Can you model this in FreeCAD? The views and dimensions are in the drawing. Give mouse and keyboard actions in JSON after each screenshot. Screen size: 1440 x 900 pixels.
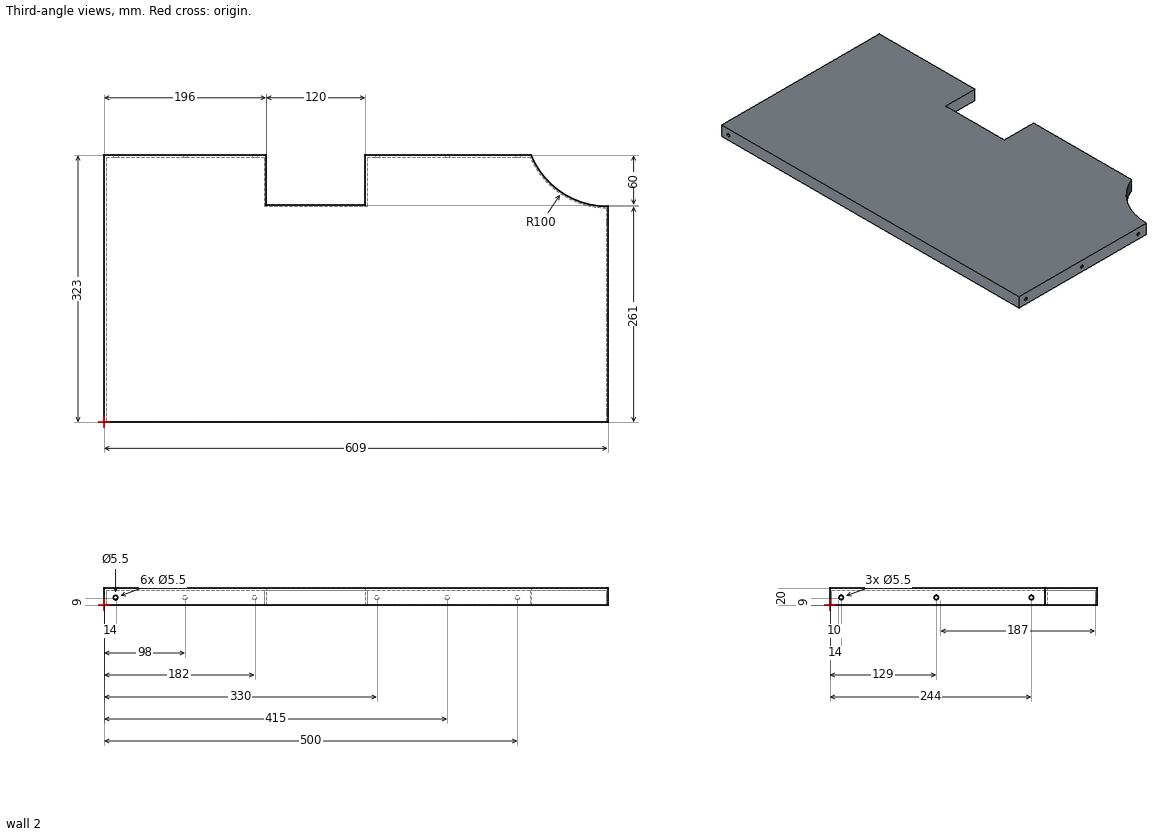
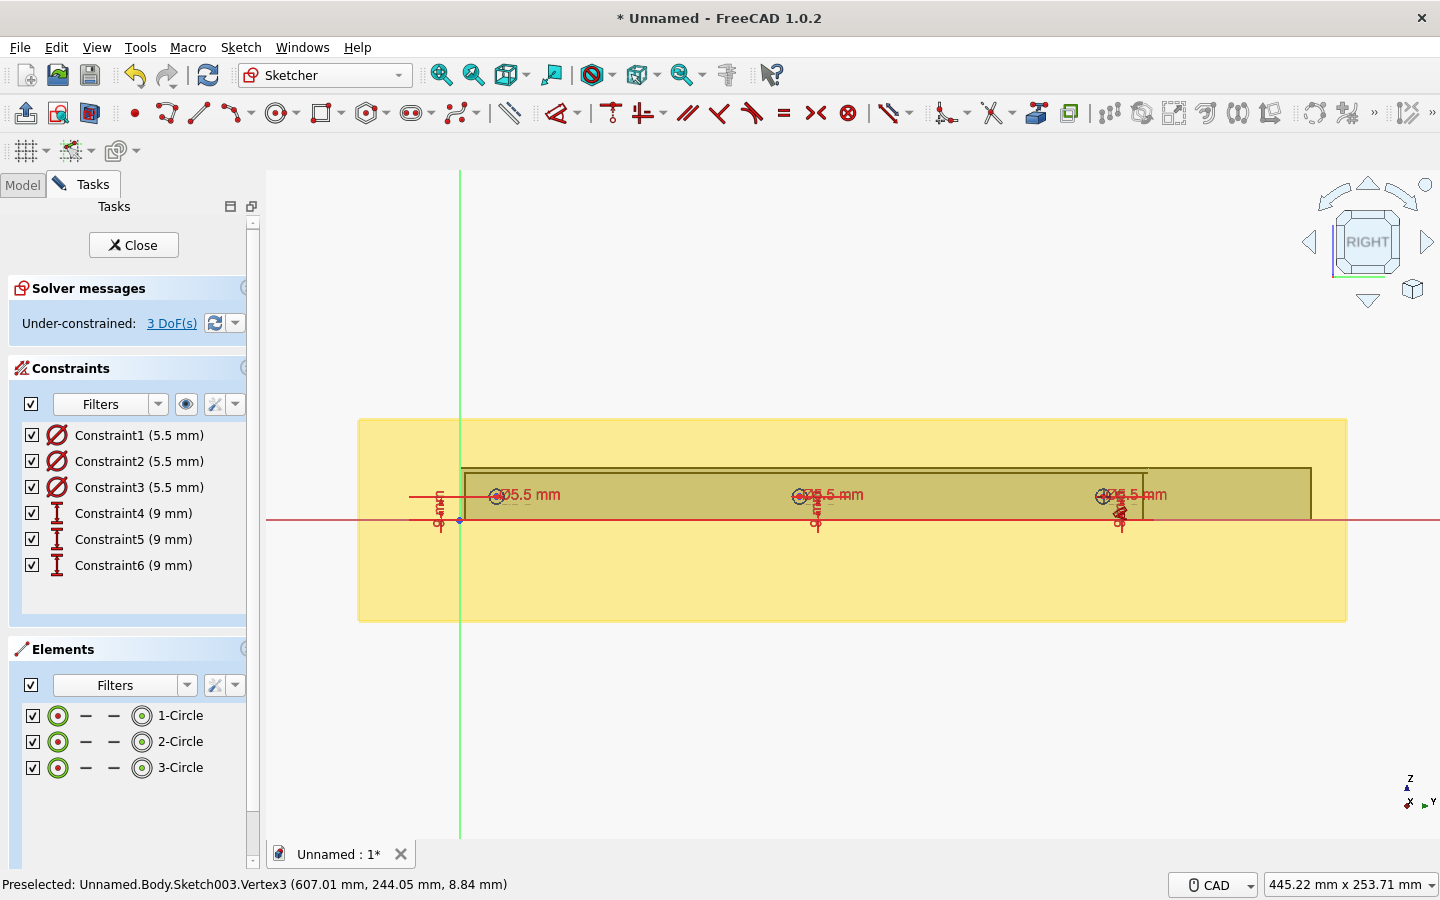
{"action": "left_click", "coordinate": [497, 497]}
{"action": "left_click", "coordinate": [478, 554]}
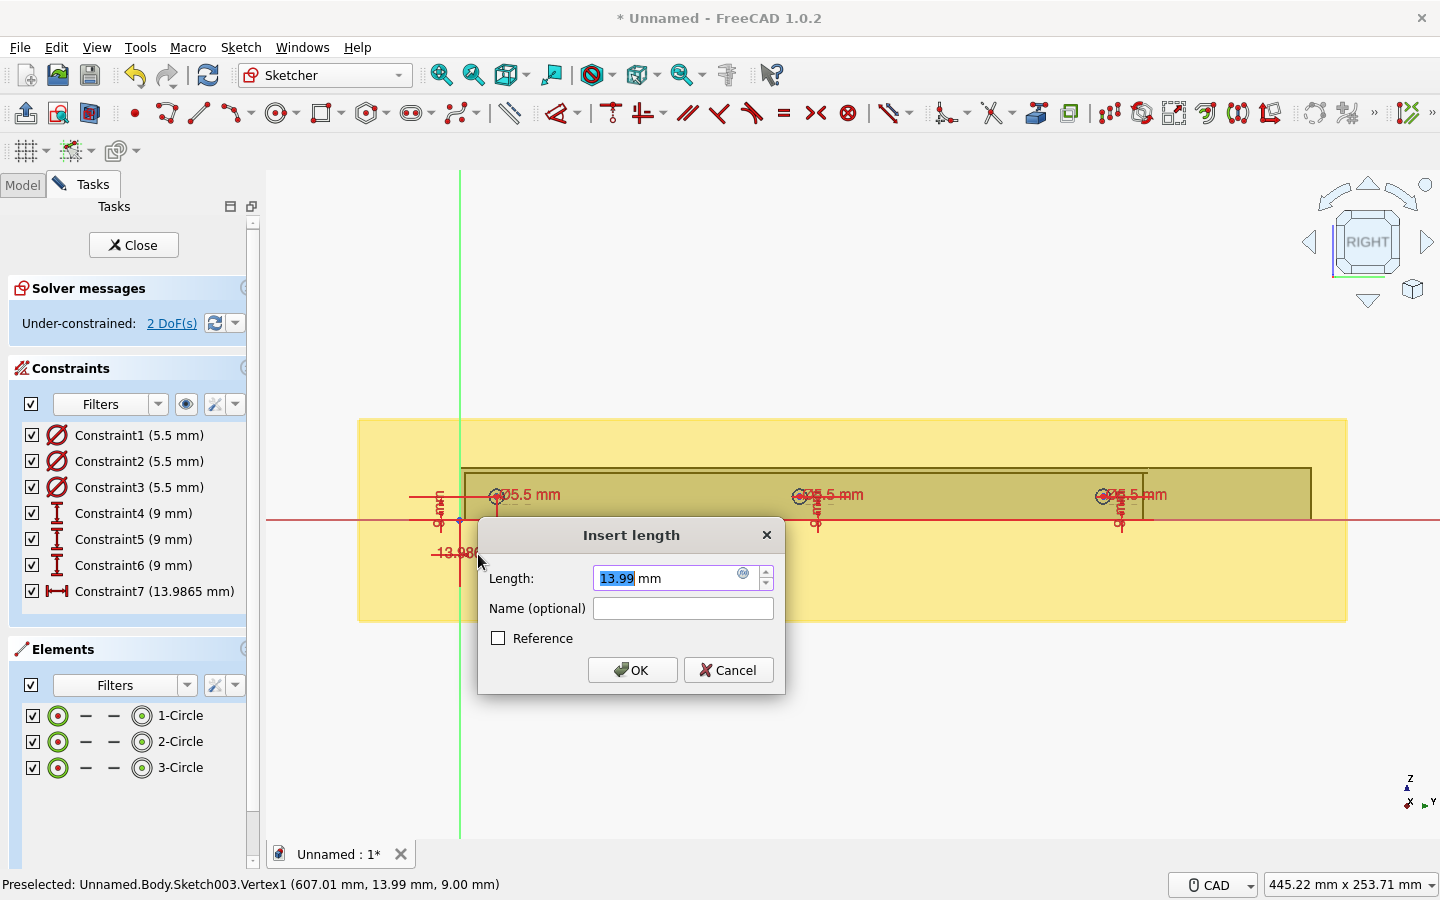
{"action": "type", "text": "14"}
{"action": "key", "text": "Return"}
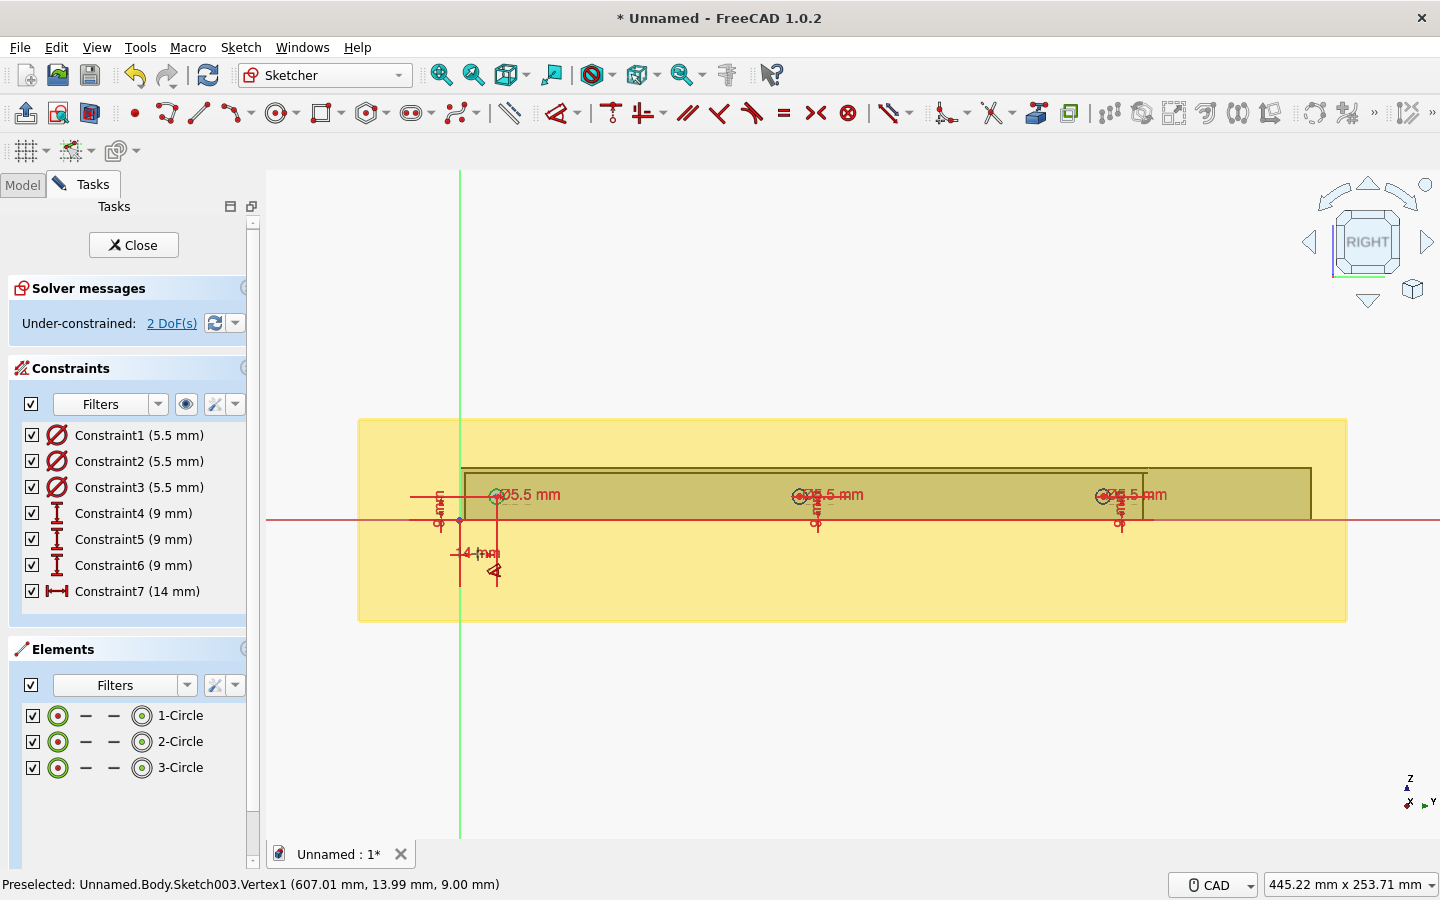
{"action": "left_click", "coordinate": [800, 497]}
{"action": "left_click", "coordinate": [630, 554]}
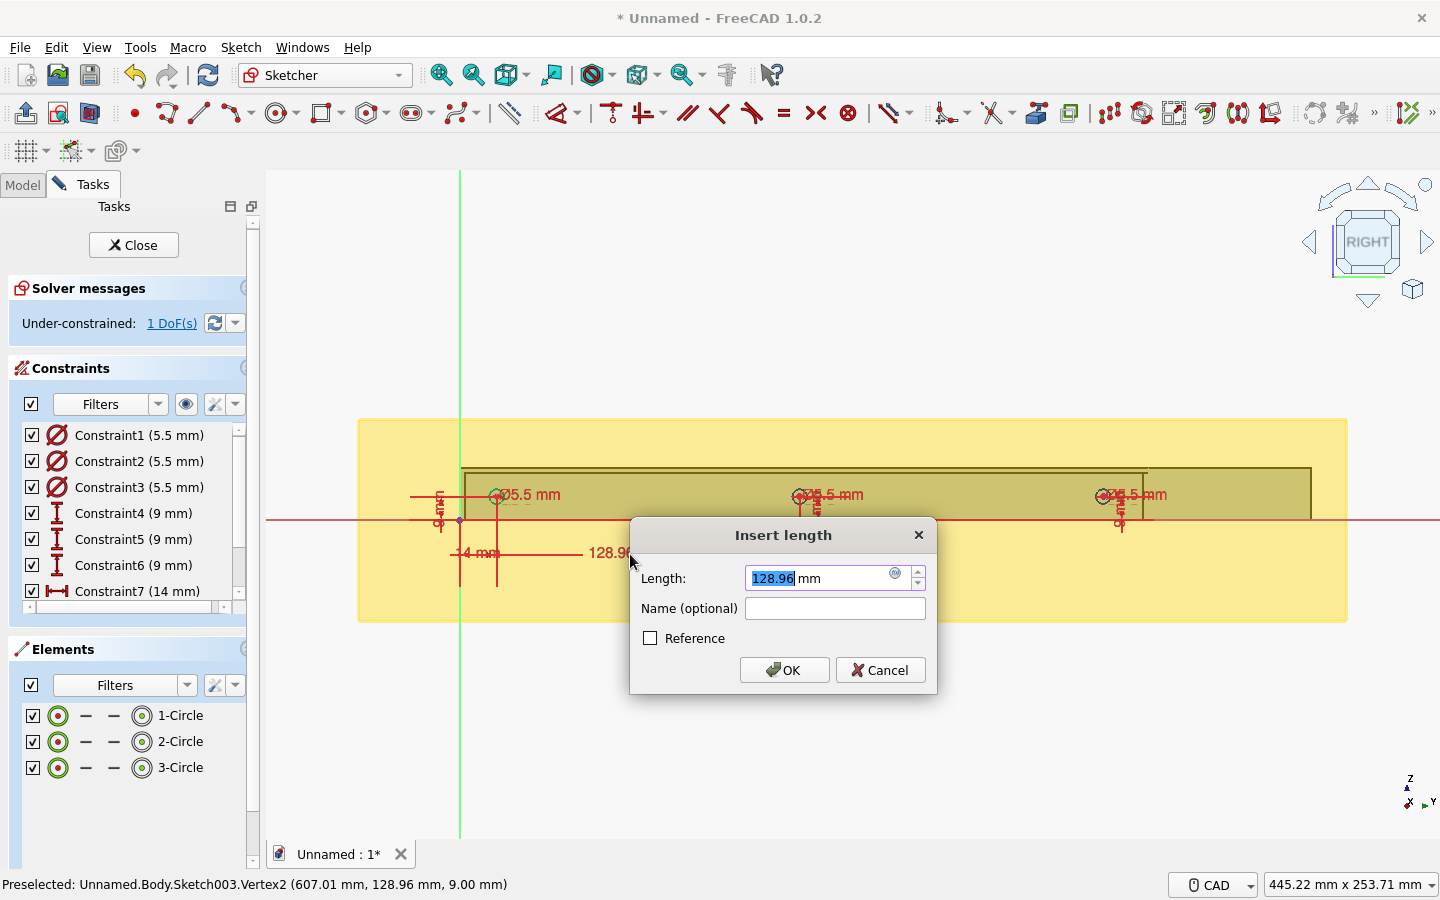
{"action": "type", "text": "129"}
{"action": "key", "text": "Return"}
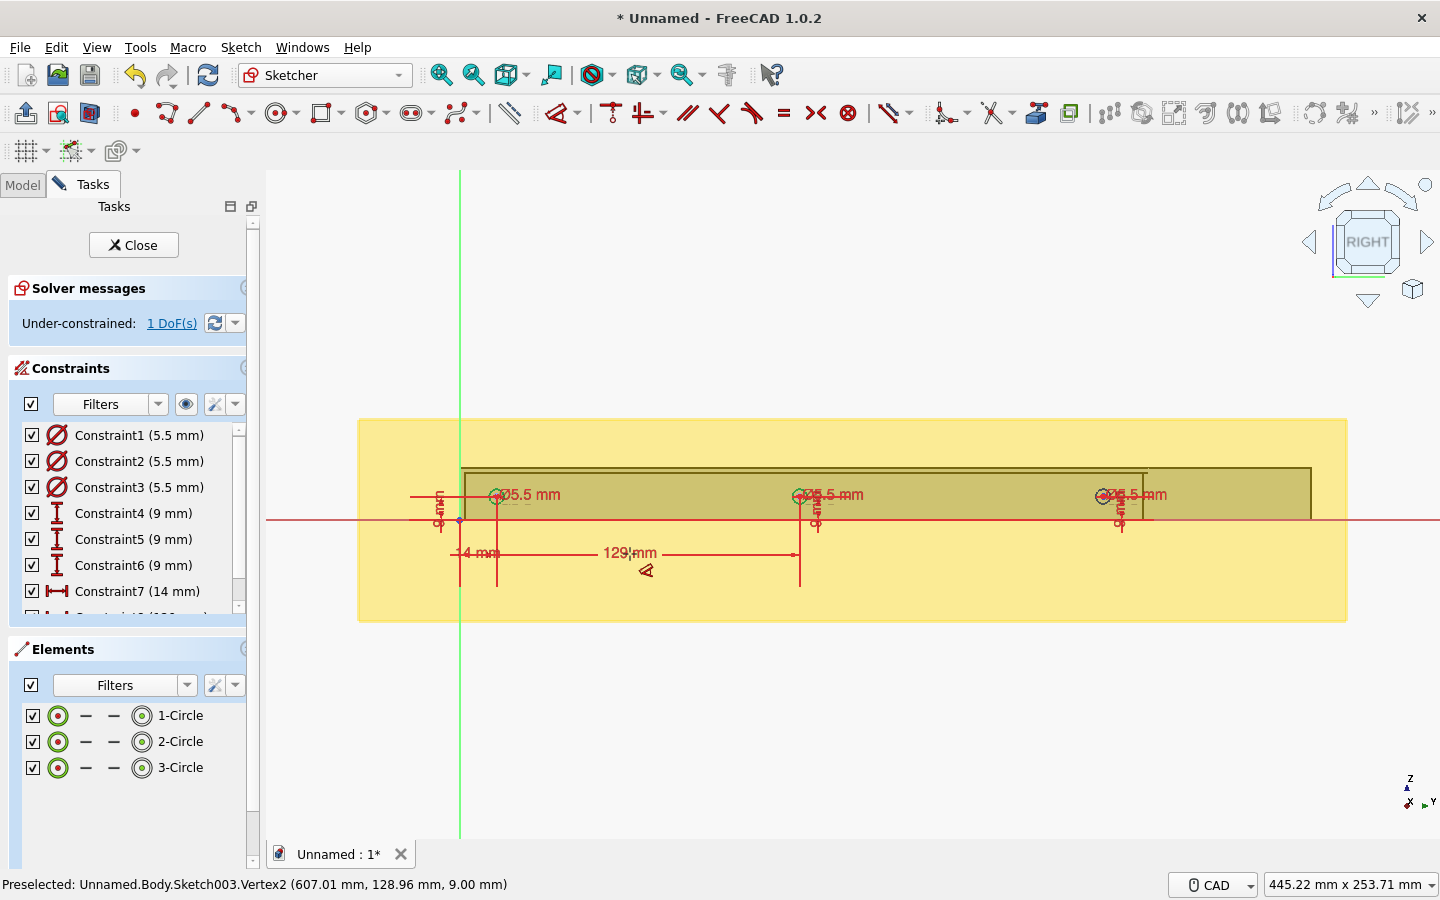
{"action": "left_click", "coordinate": [1103, 497]}
{"action": "left_click", "coordinate": [781, 554]}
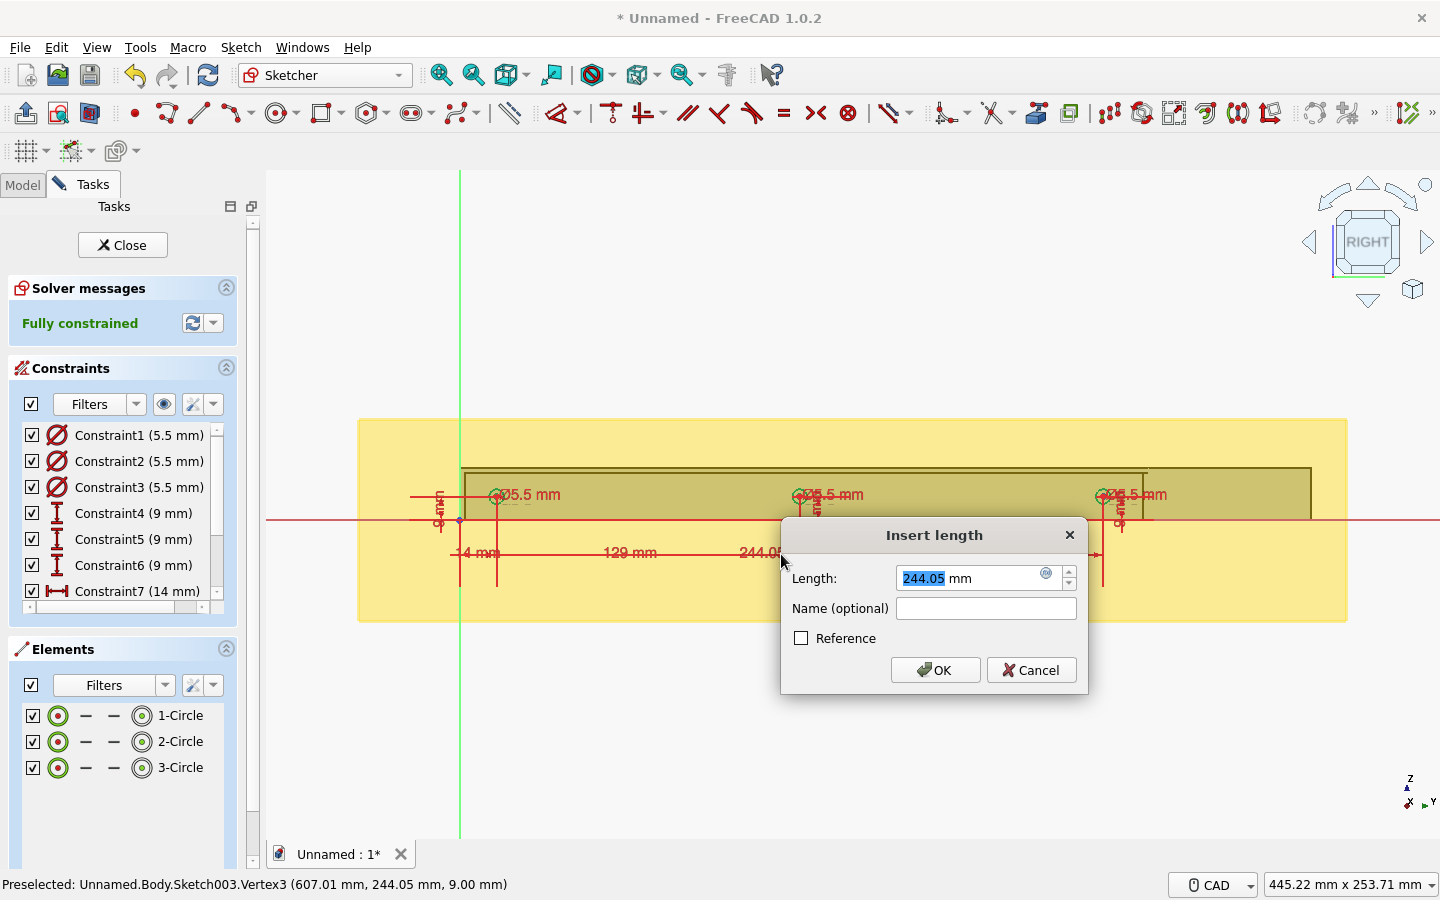
{"action": "type", "text": "244"}
{"action": "key", "text": "Return"}
{"action": "key", "text": "Escape"}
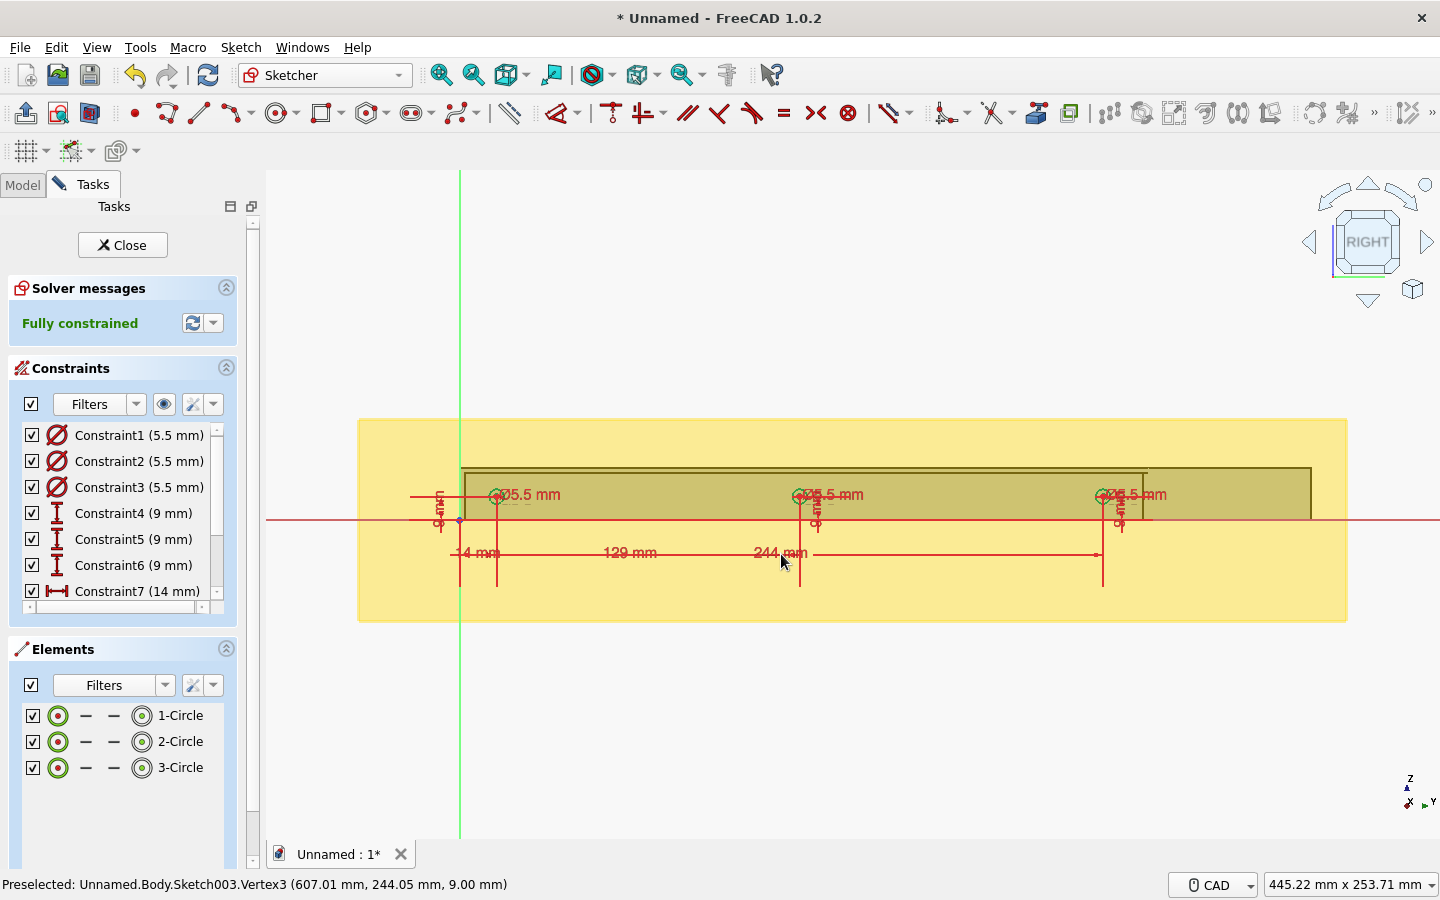
{"action": "left_click", "coordinate": [123, 245]}